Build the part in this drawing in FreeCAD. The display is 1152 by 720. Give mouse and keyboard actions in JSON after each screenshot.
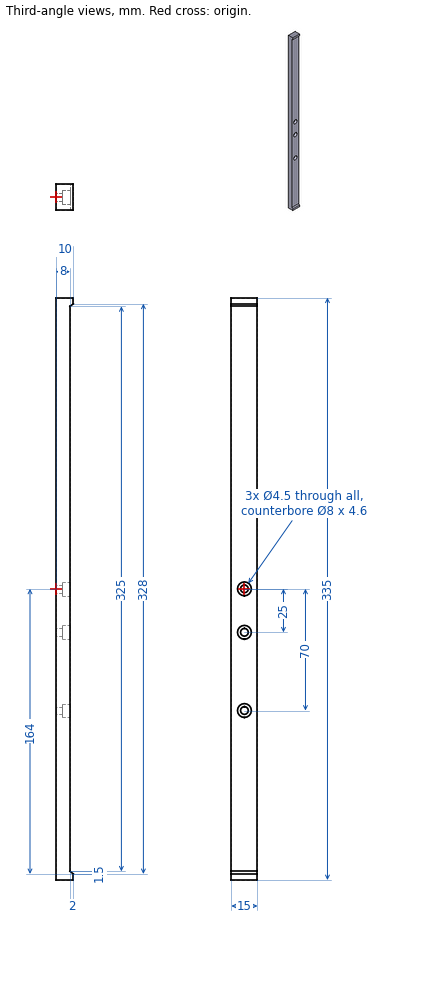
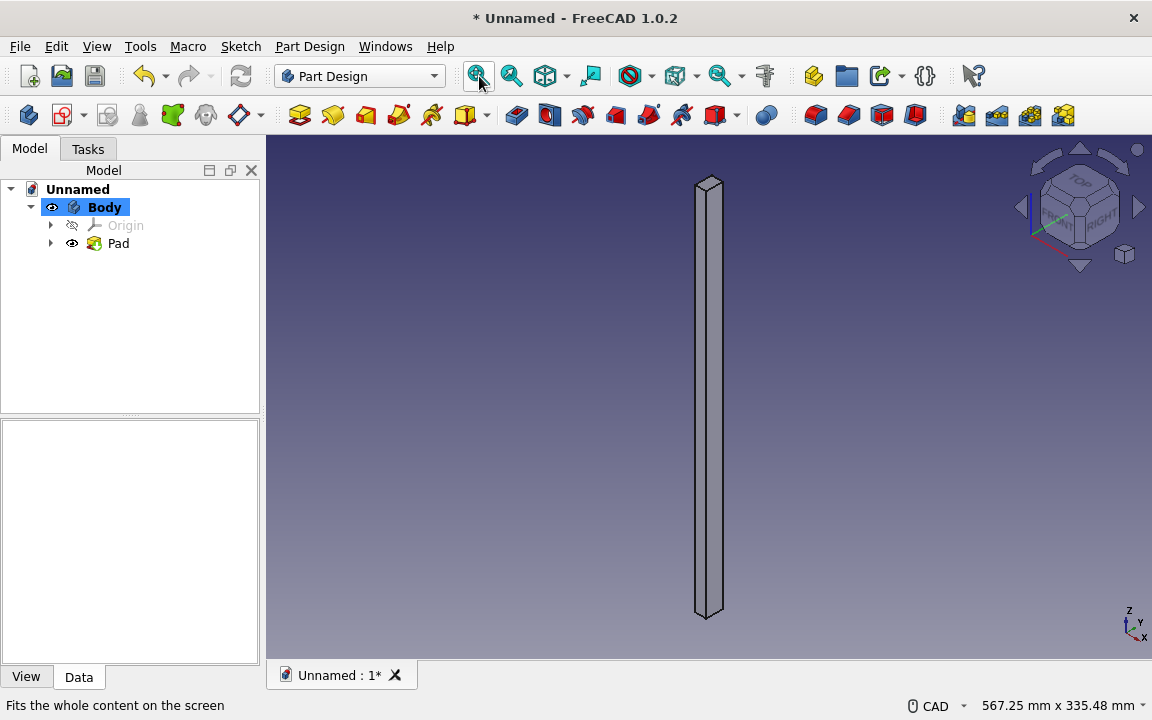
{"action": "key", "text": "1"}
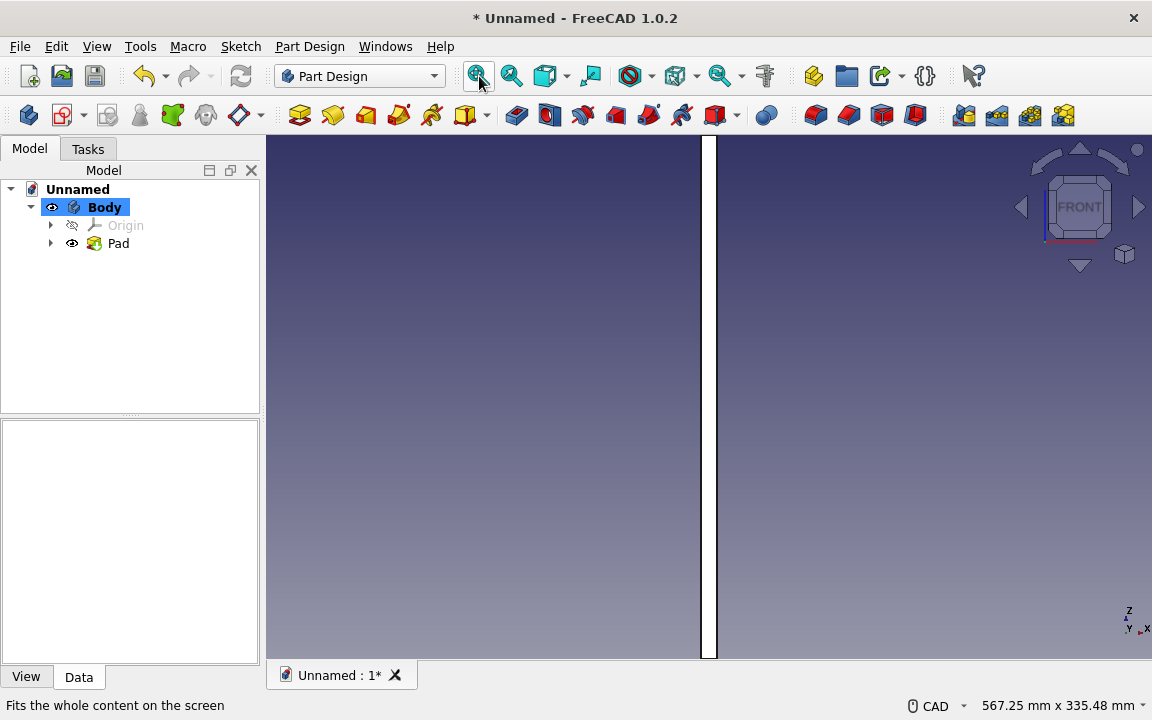
{"action": "left_click", "coordinate": [479, 76]}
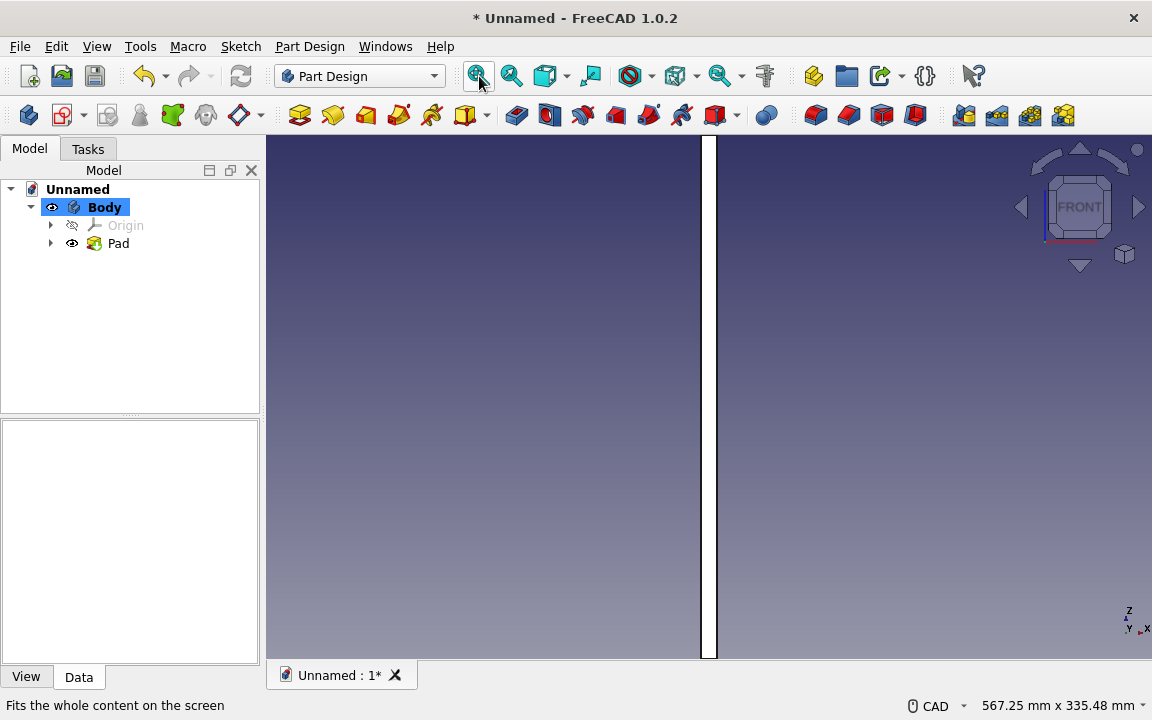
{"action": "key", "text": "6"}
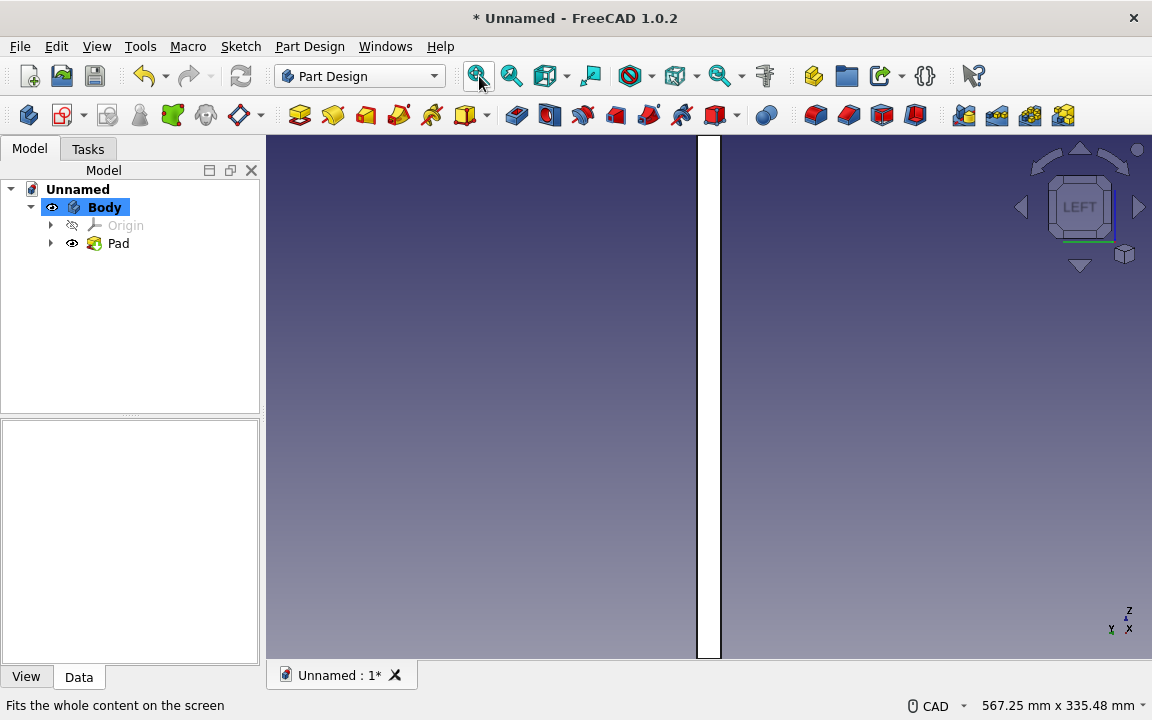
{"action": "left_click", "coordinate": [479, 76]}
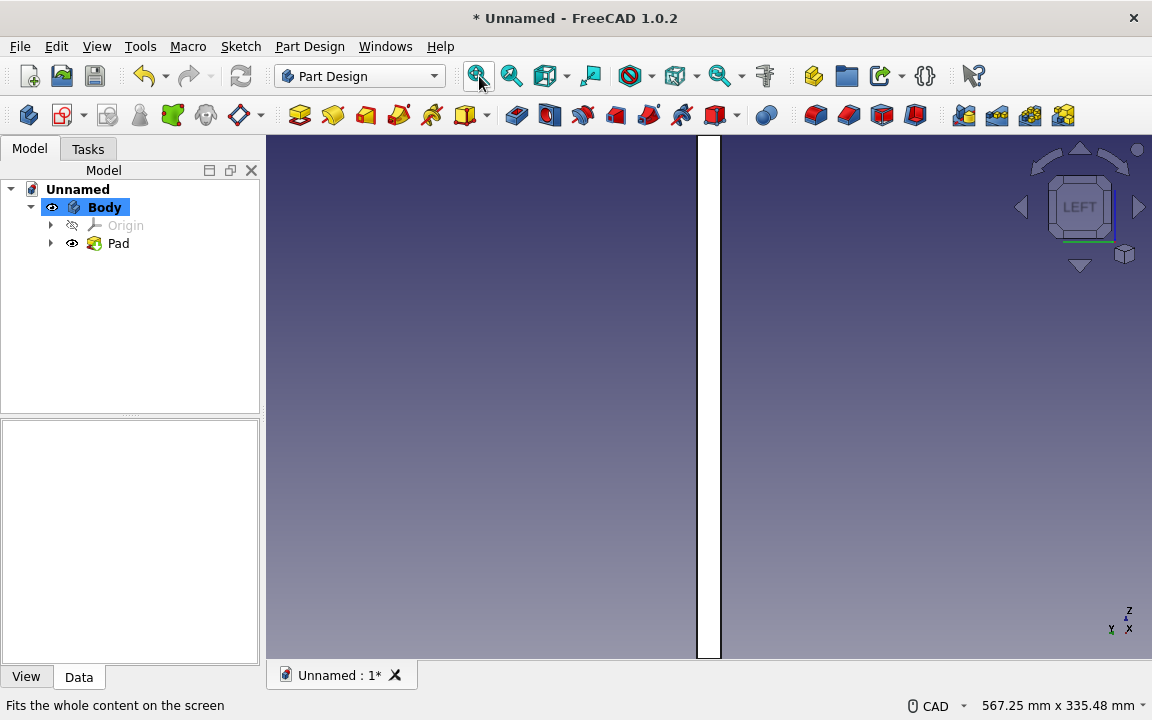
{"action": "left_click", "coordinate": [51, 225]}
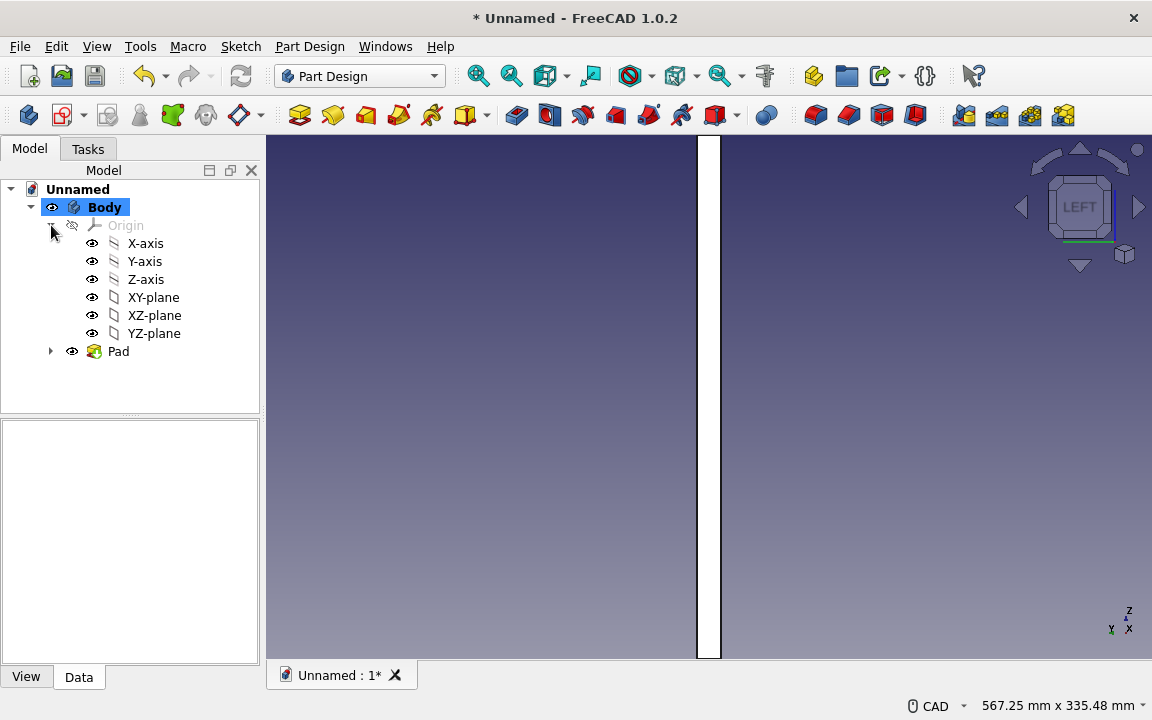
{"action": "left_click", "coordinate": [137, 315]}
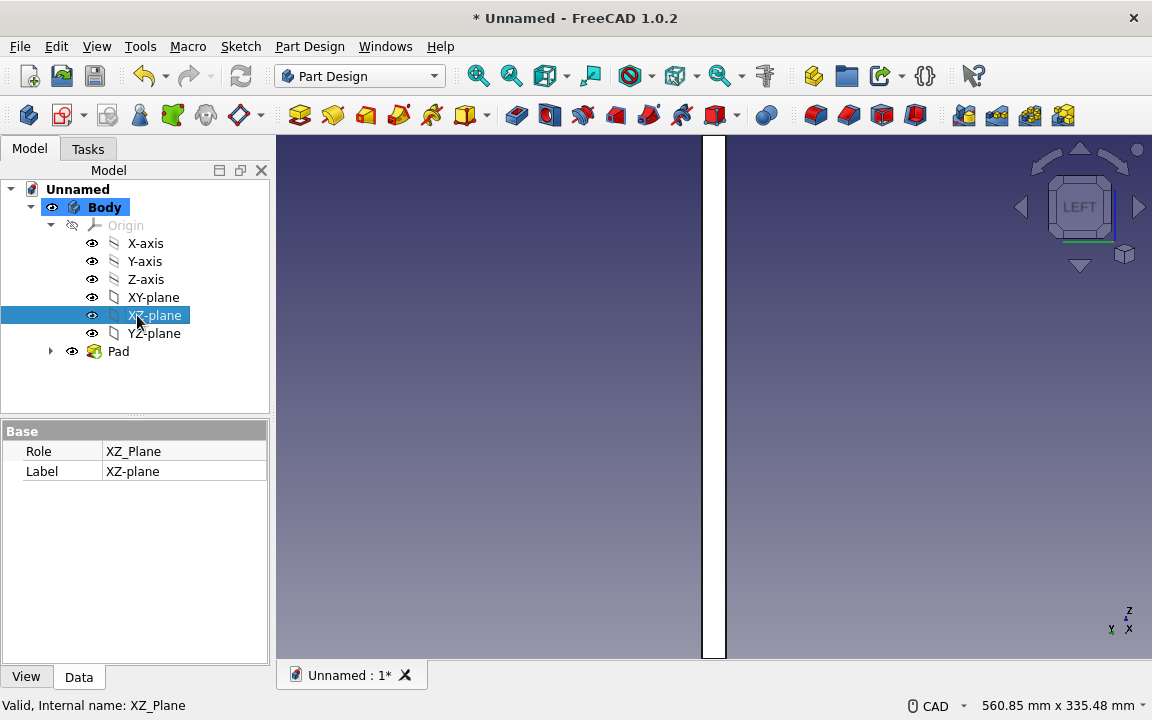
{"action": "left_click", "coordinate": [238, 116]}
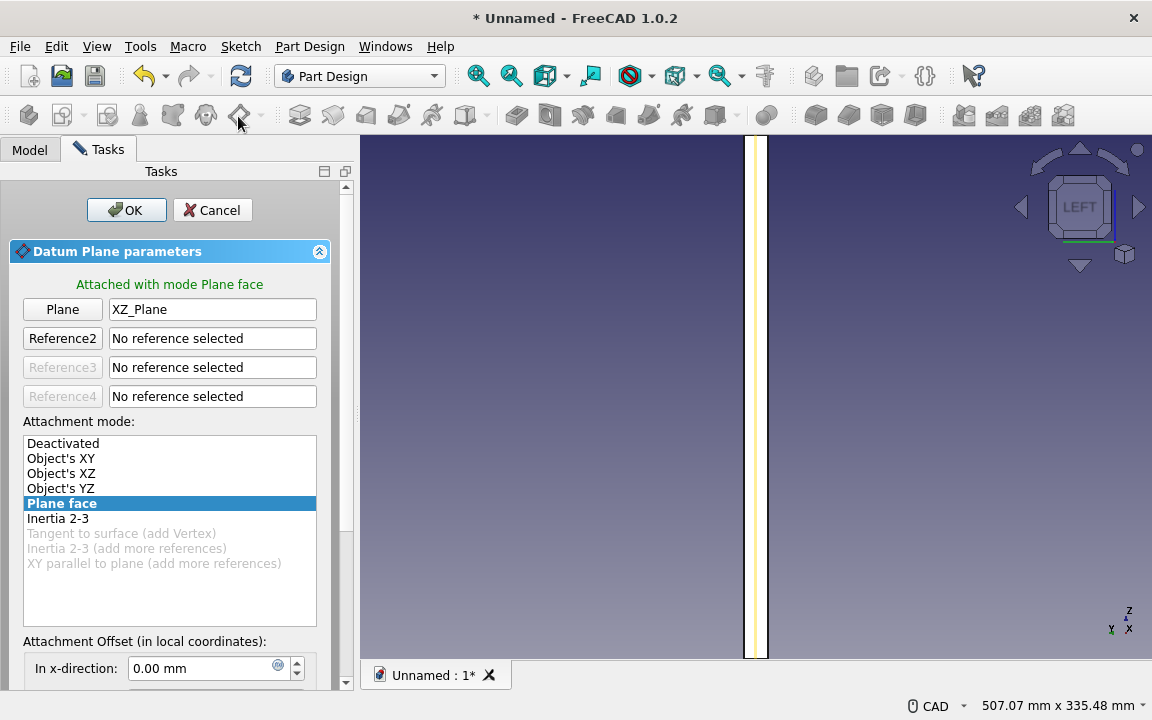
{"action": "scroll", "coordinate": [346, 436], "scroll_direction": "down", "scroll_amount": 2}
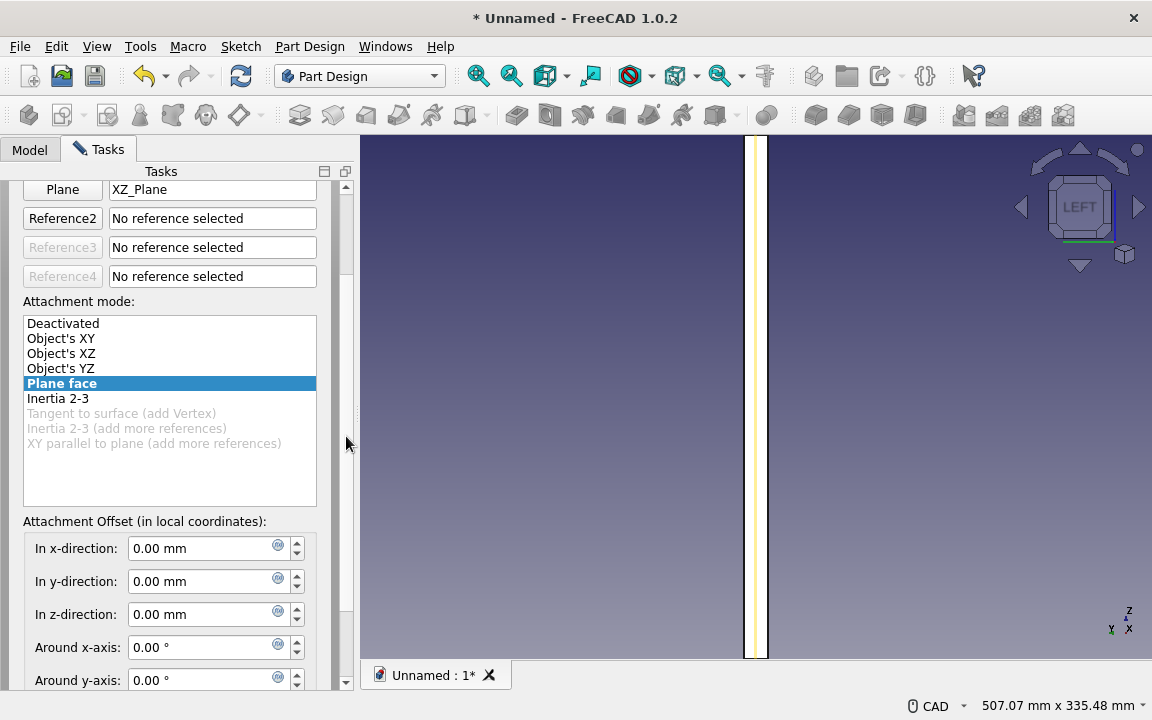
{"action": "triple_click", "coordinate": [210, 614]}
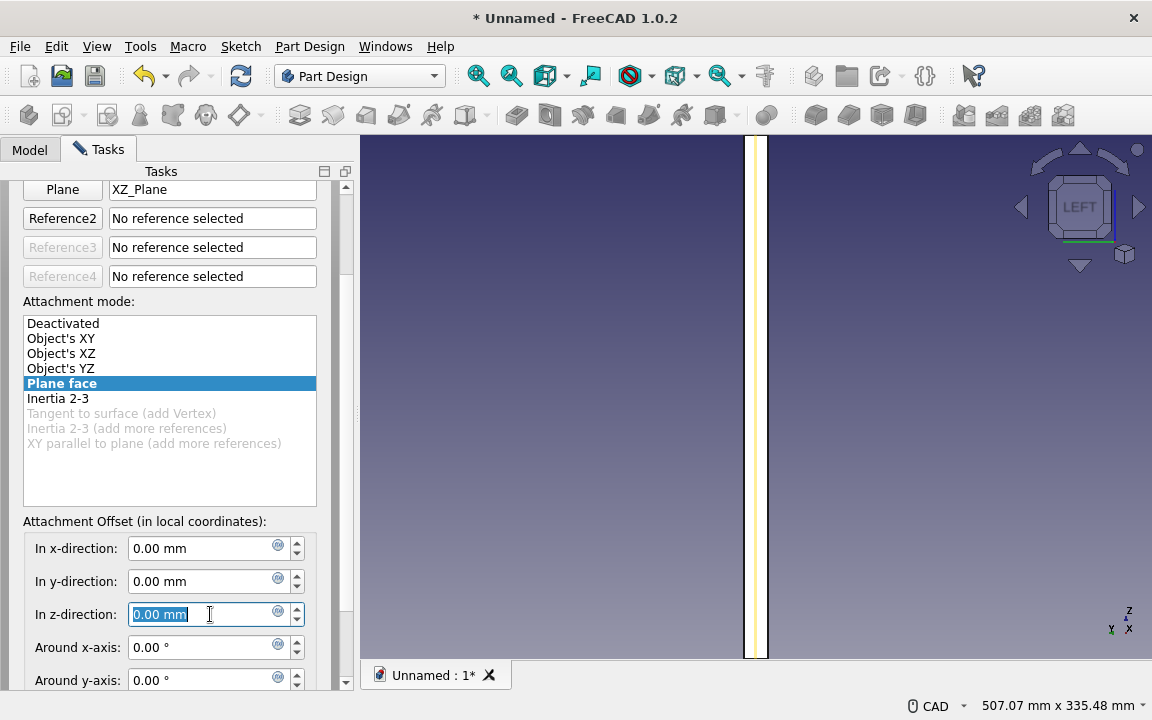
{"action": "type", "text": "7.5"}
{"action": "key", "text": "Tab"}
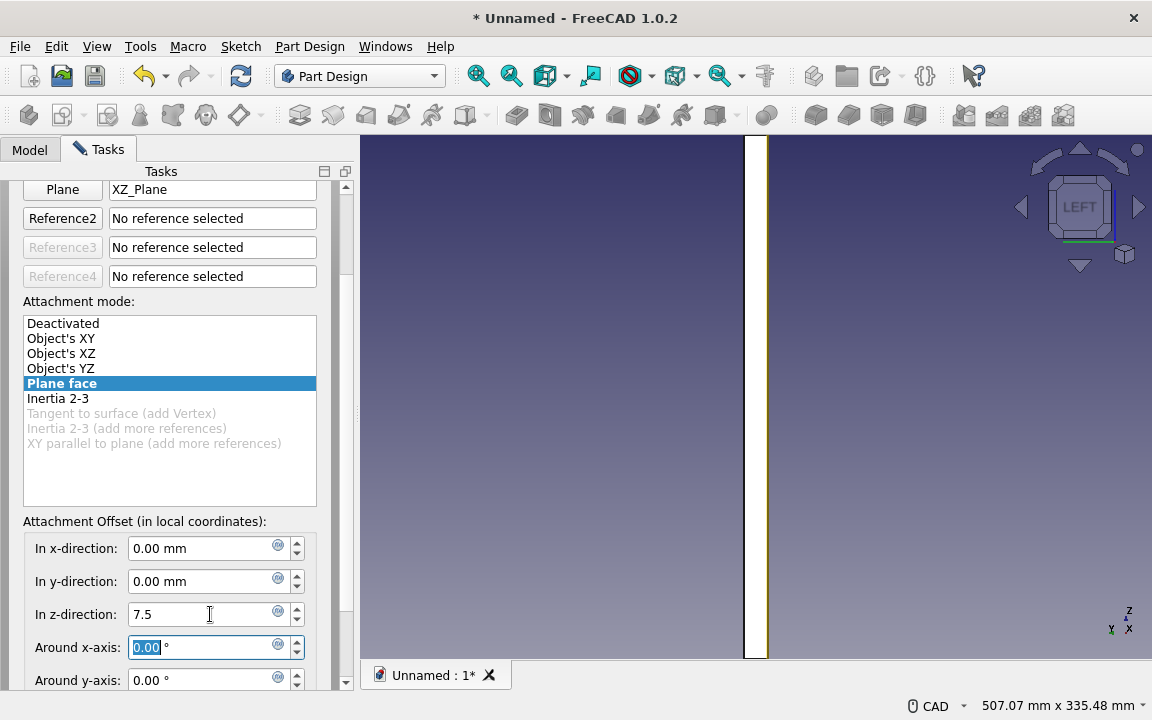
{"action": "scroll", "coordinate": [346, 436], "scroll_direction": "up", "scroll_amount": 3}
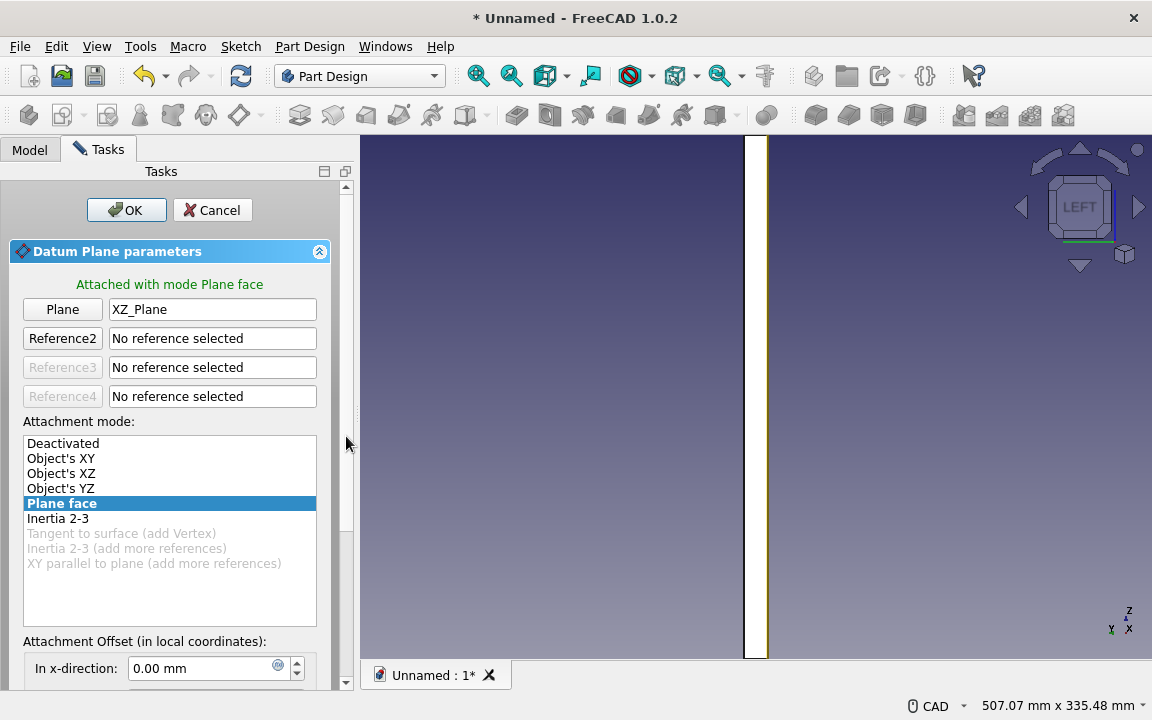
{"action": "left_click", "coordinate": [127, 210]}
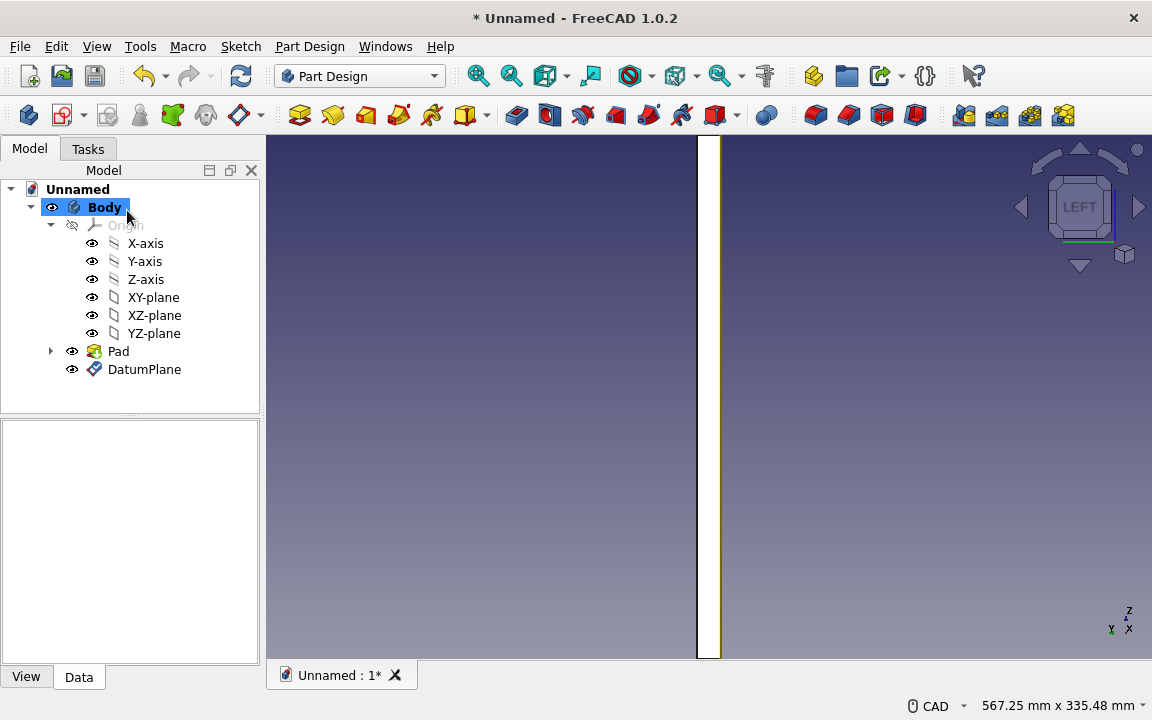
{"action": "left_click", "coordinate": [117, 369]}